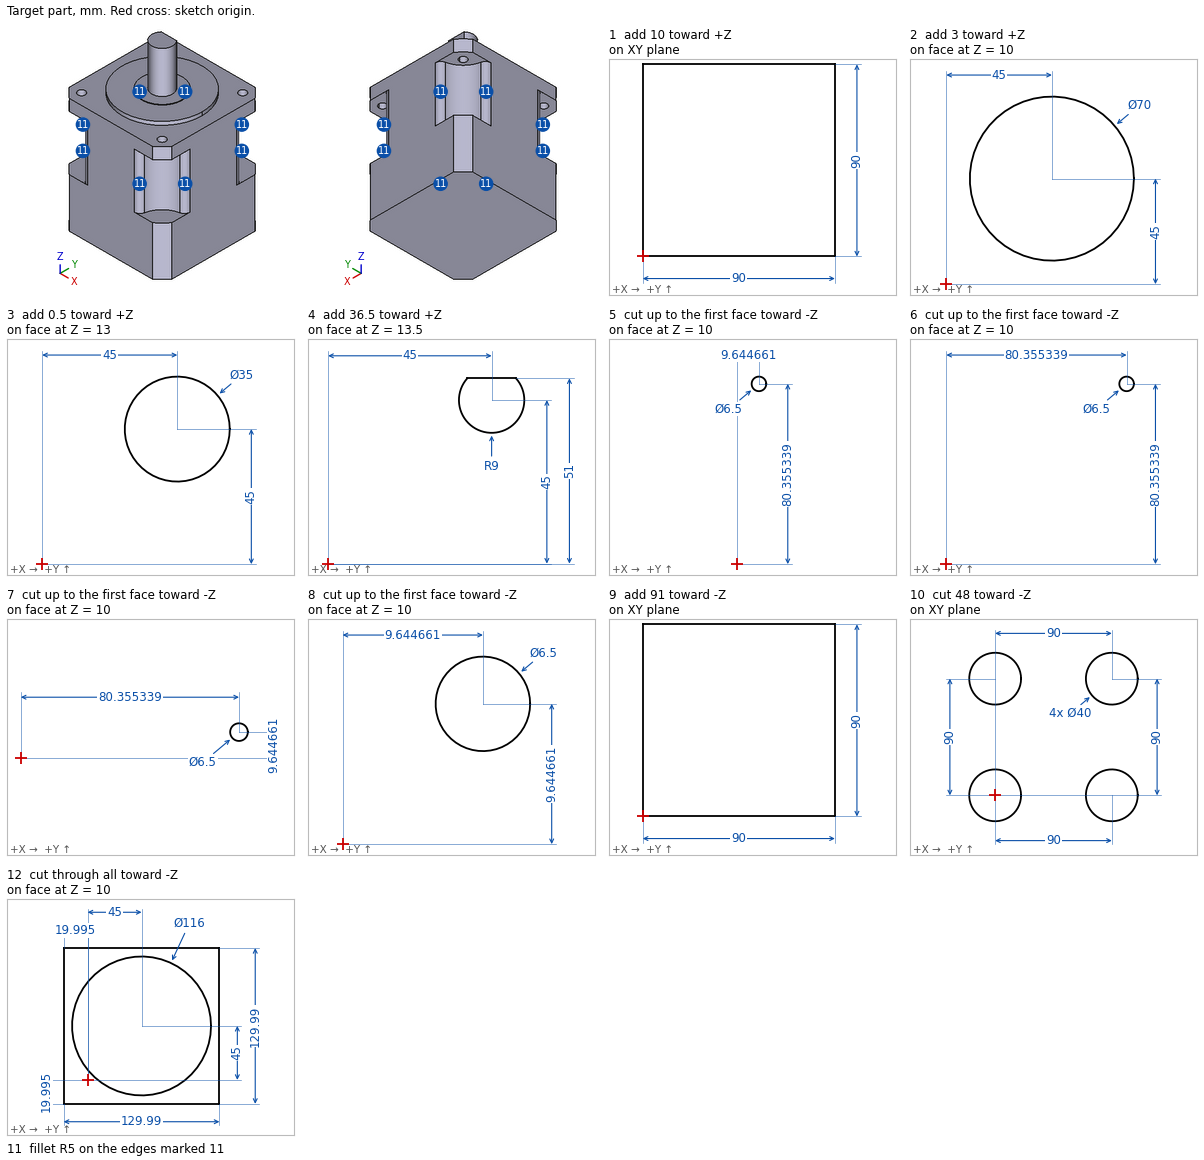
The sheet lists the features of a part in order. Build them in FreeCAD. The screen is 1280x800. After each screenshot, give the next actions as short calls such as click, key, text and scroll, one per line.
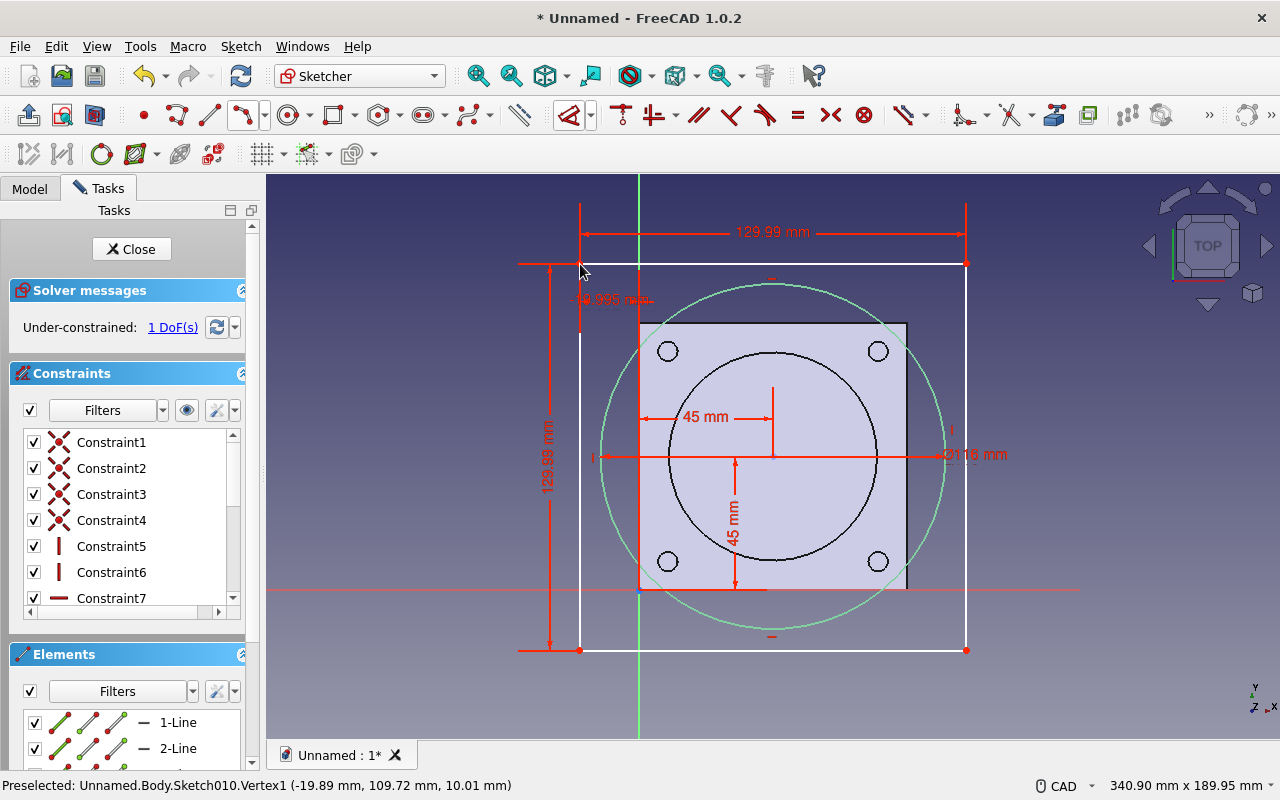
click(580, 651)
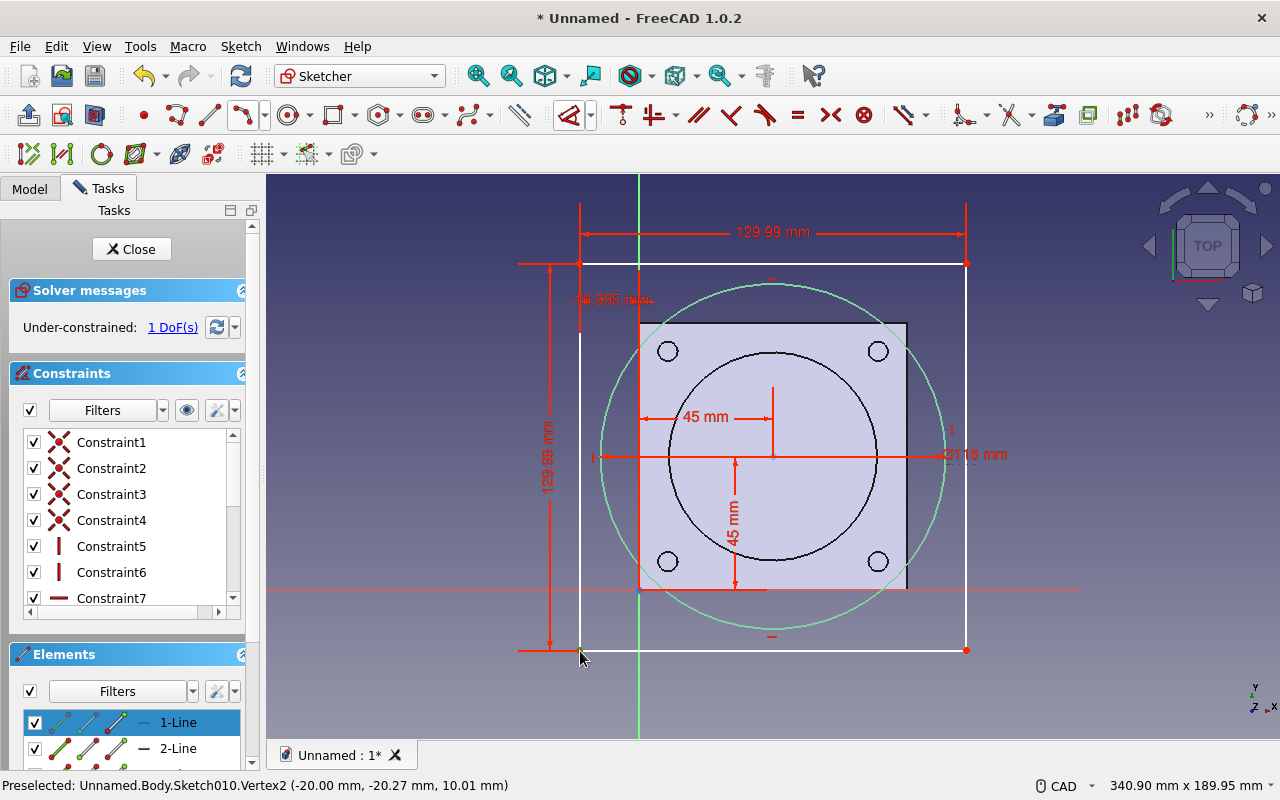
key(i)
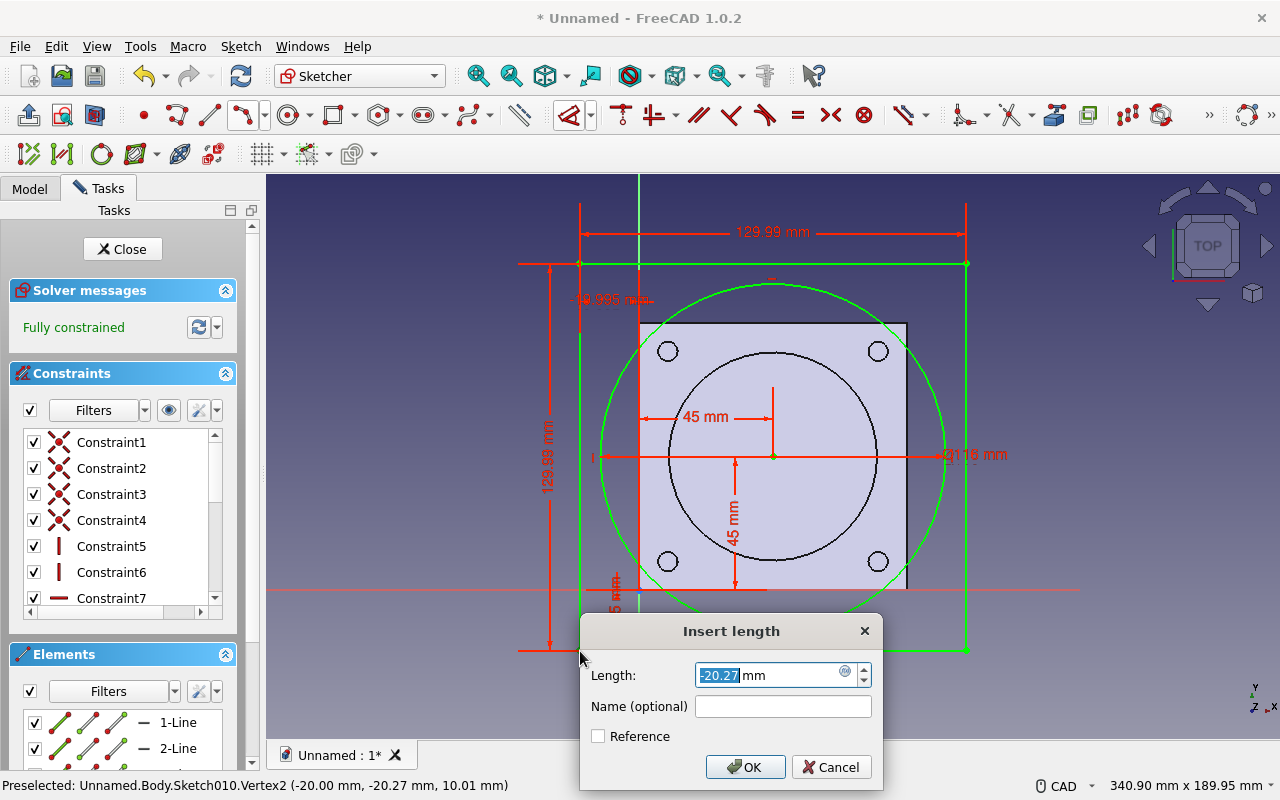
text(-19.995)
key(Return)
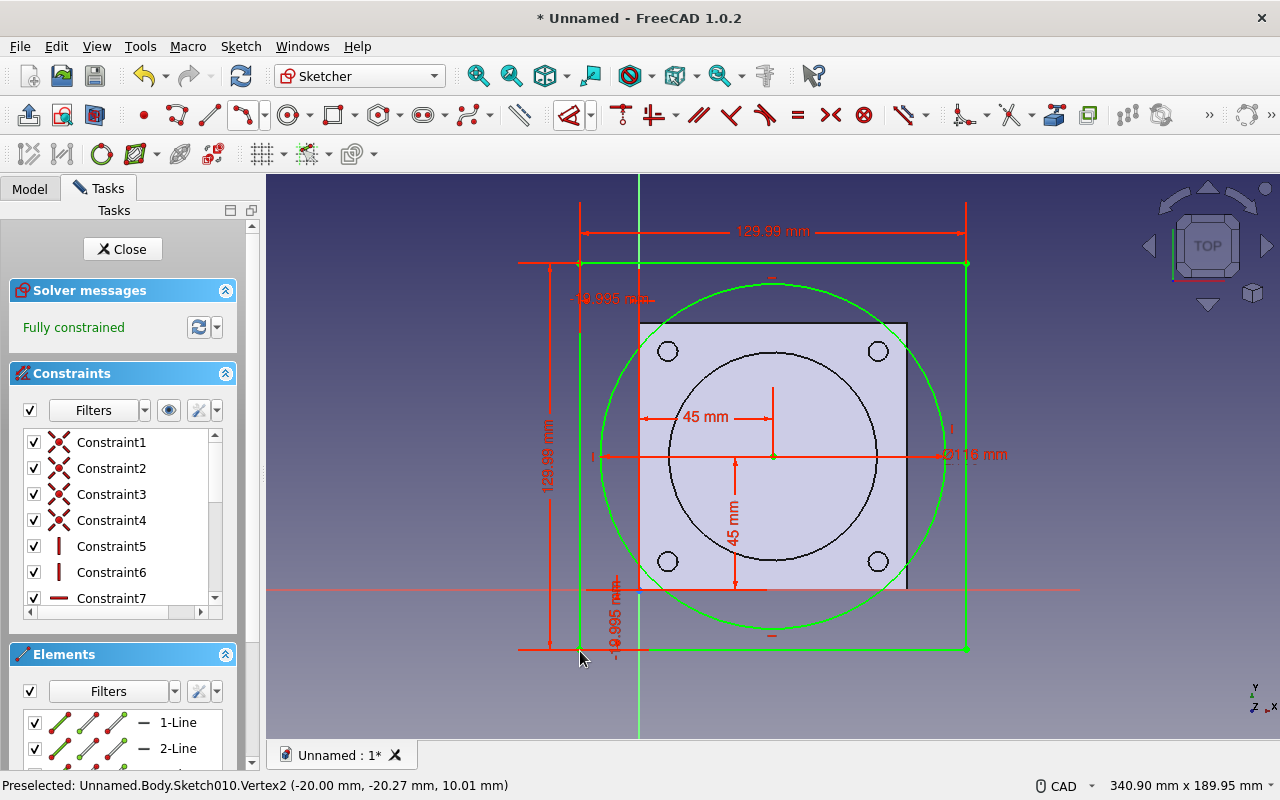
click(123, 249)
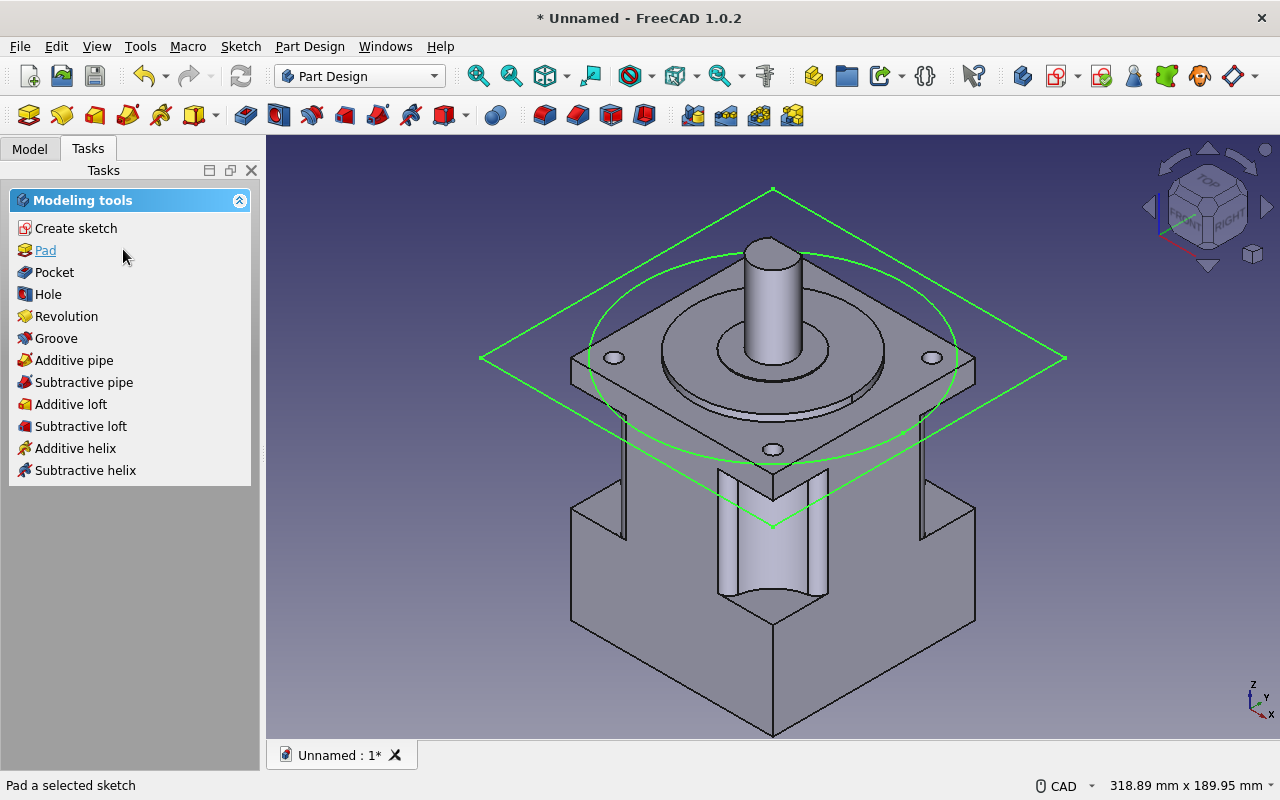
click(246, 116)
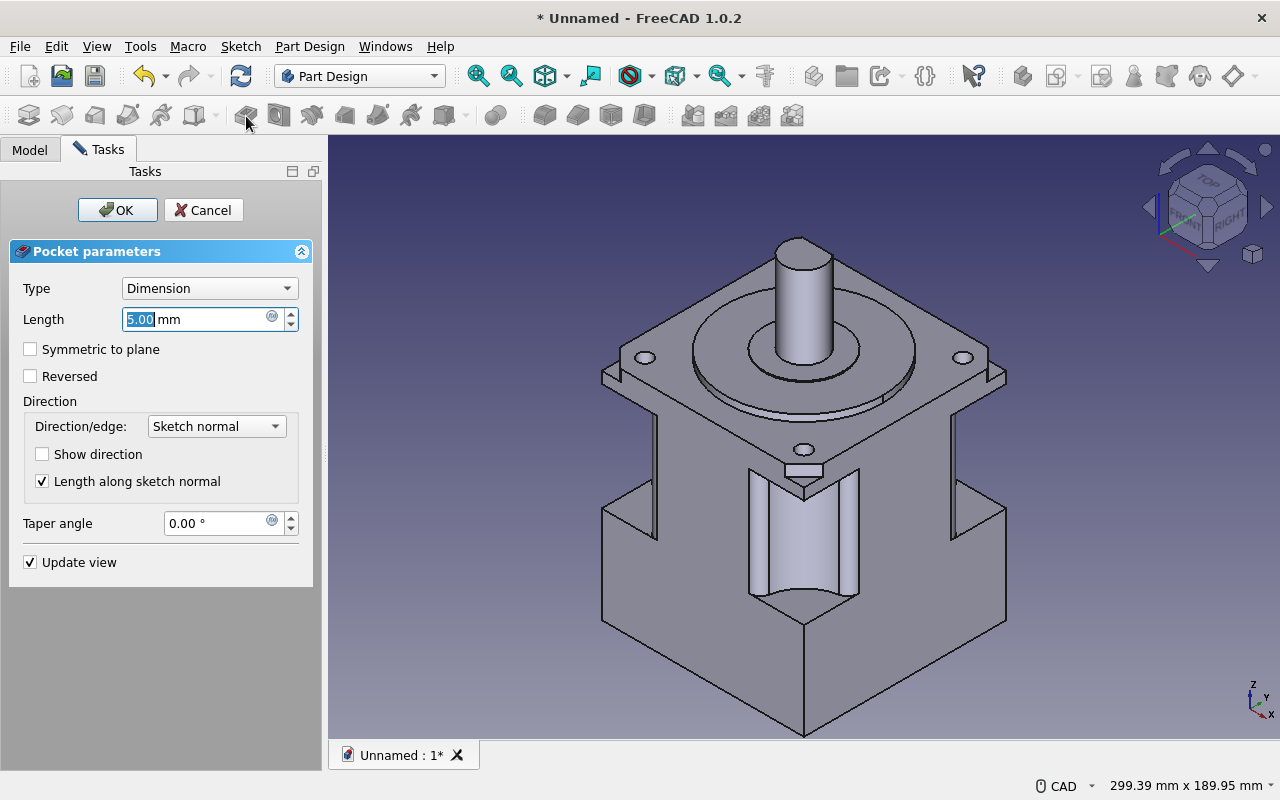
click(210, 288)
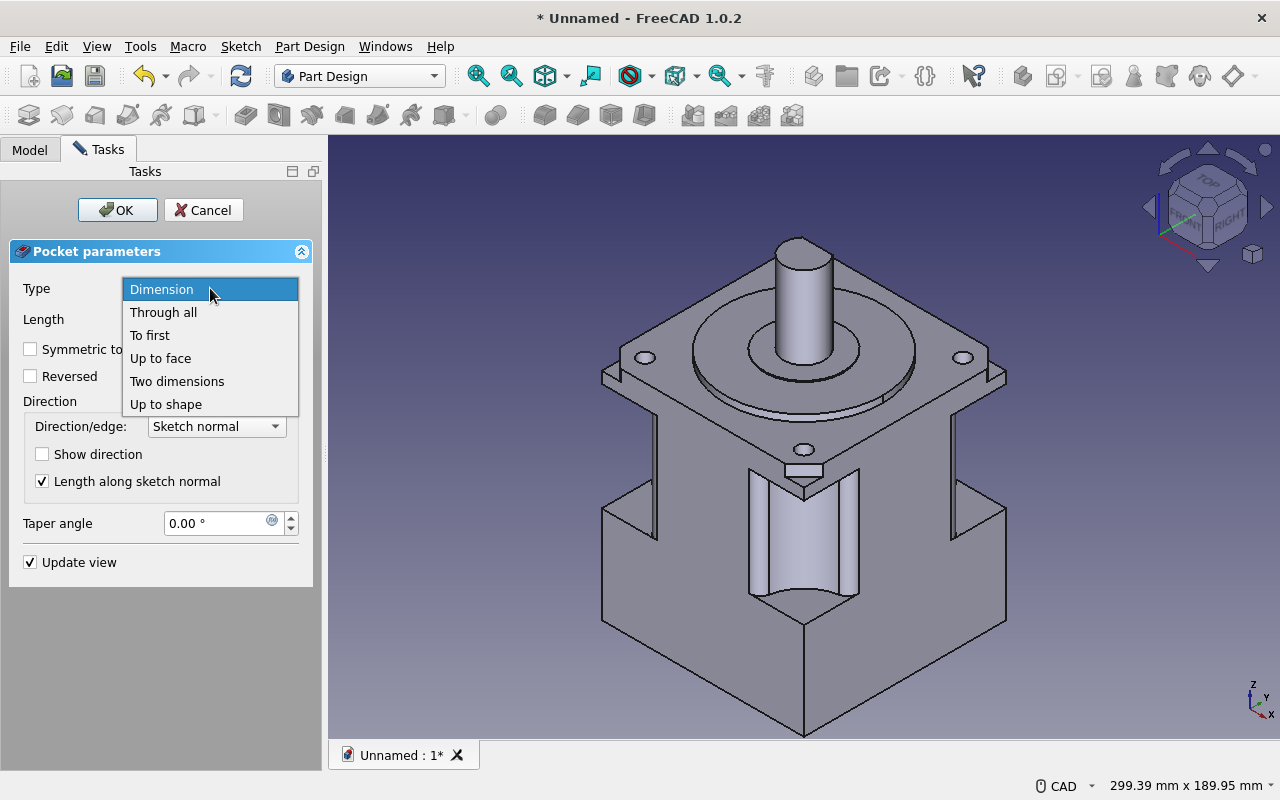
click(208, 312)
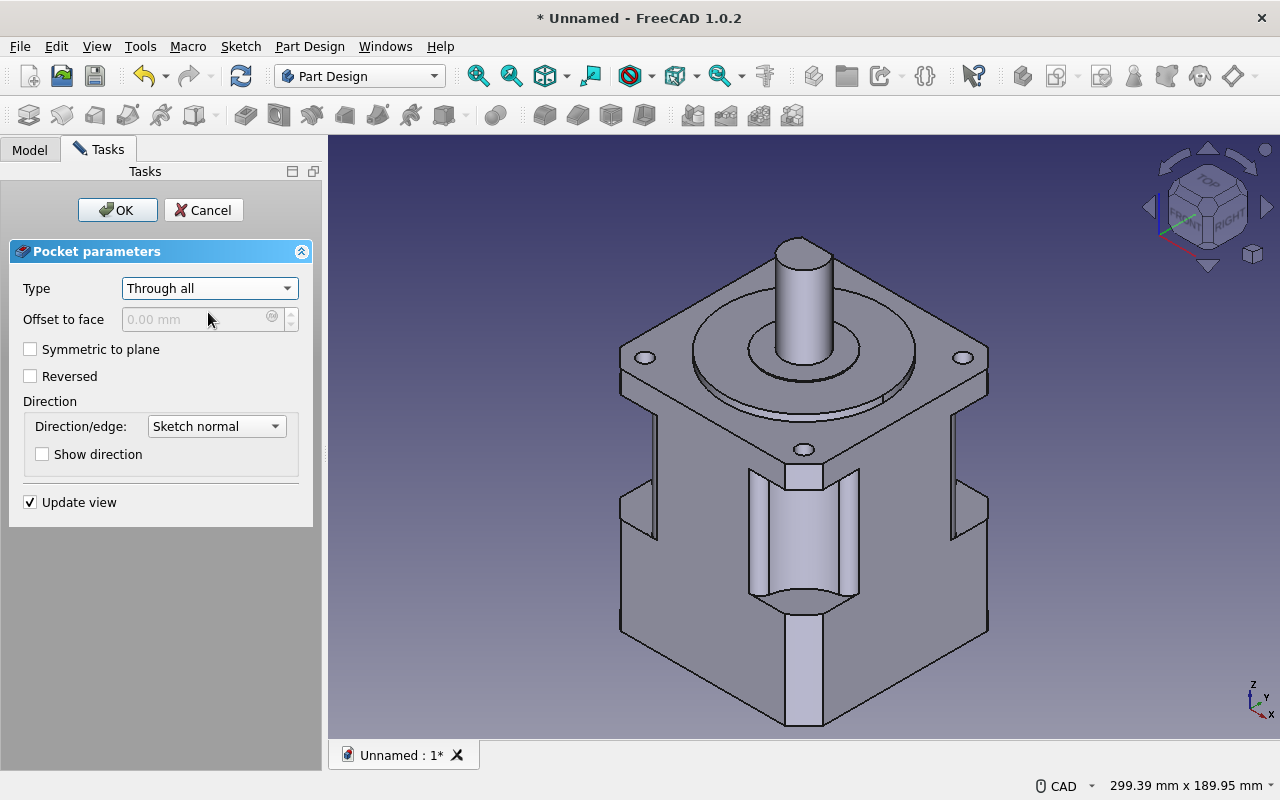
click(118, 210)